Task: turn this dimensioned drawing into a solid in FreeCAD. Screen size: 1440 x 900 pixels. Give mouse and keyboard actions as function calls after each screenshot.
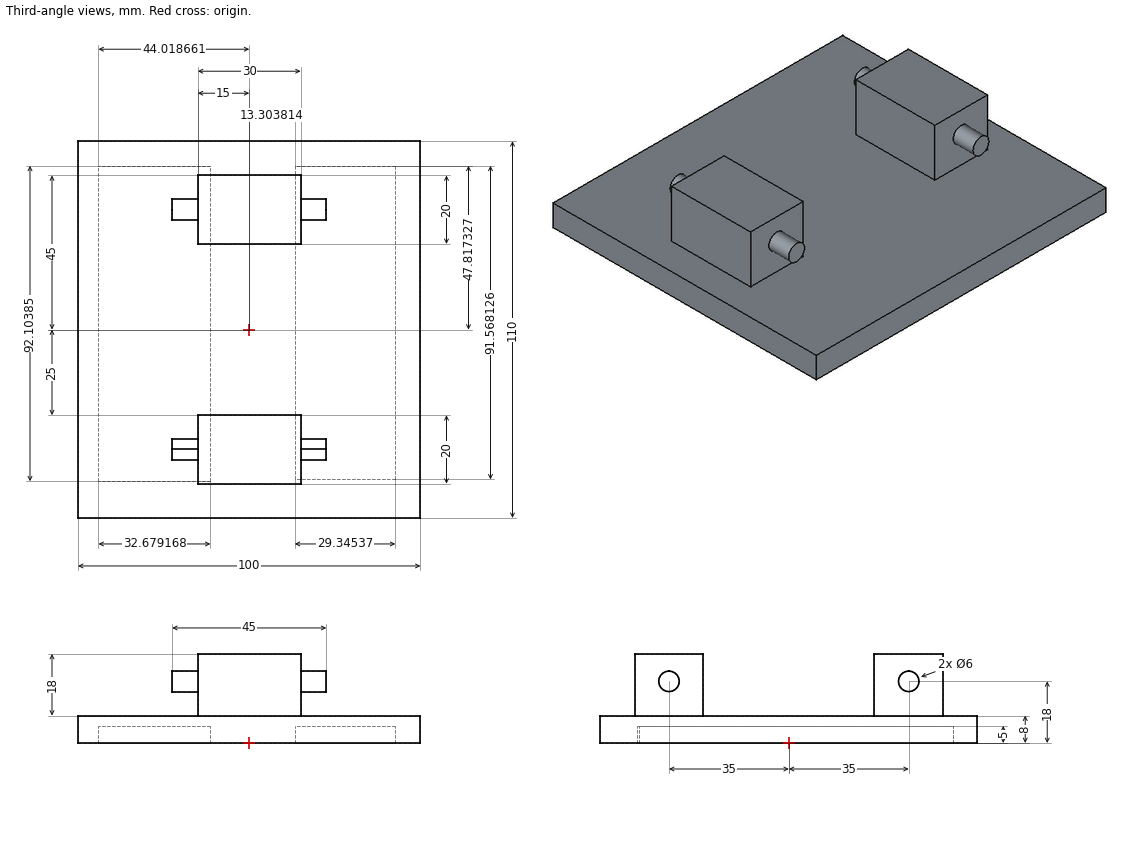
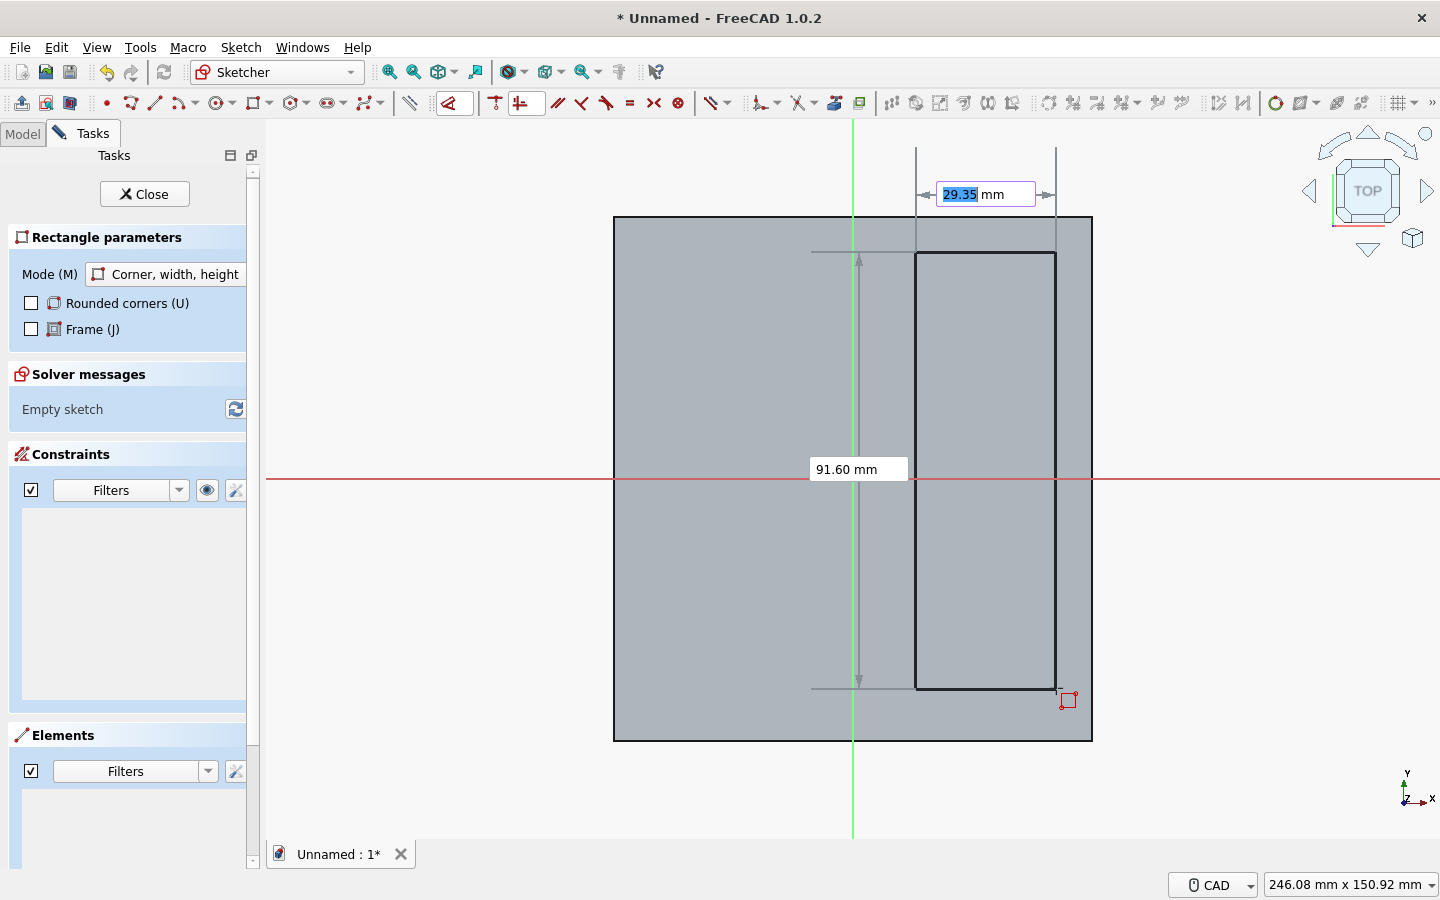
text(29.34537)
key(Tab)
text(91.568126)
key(Return)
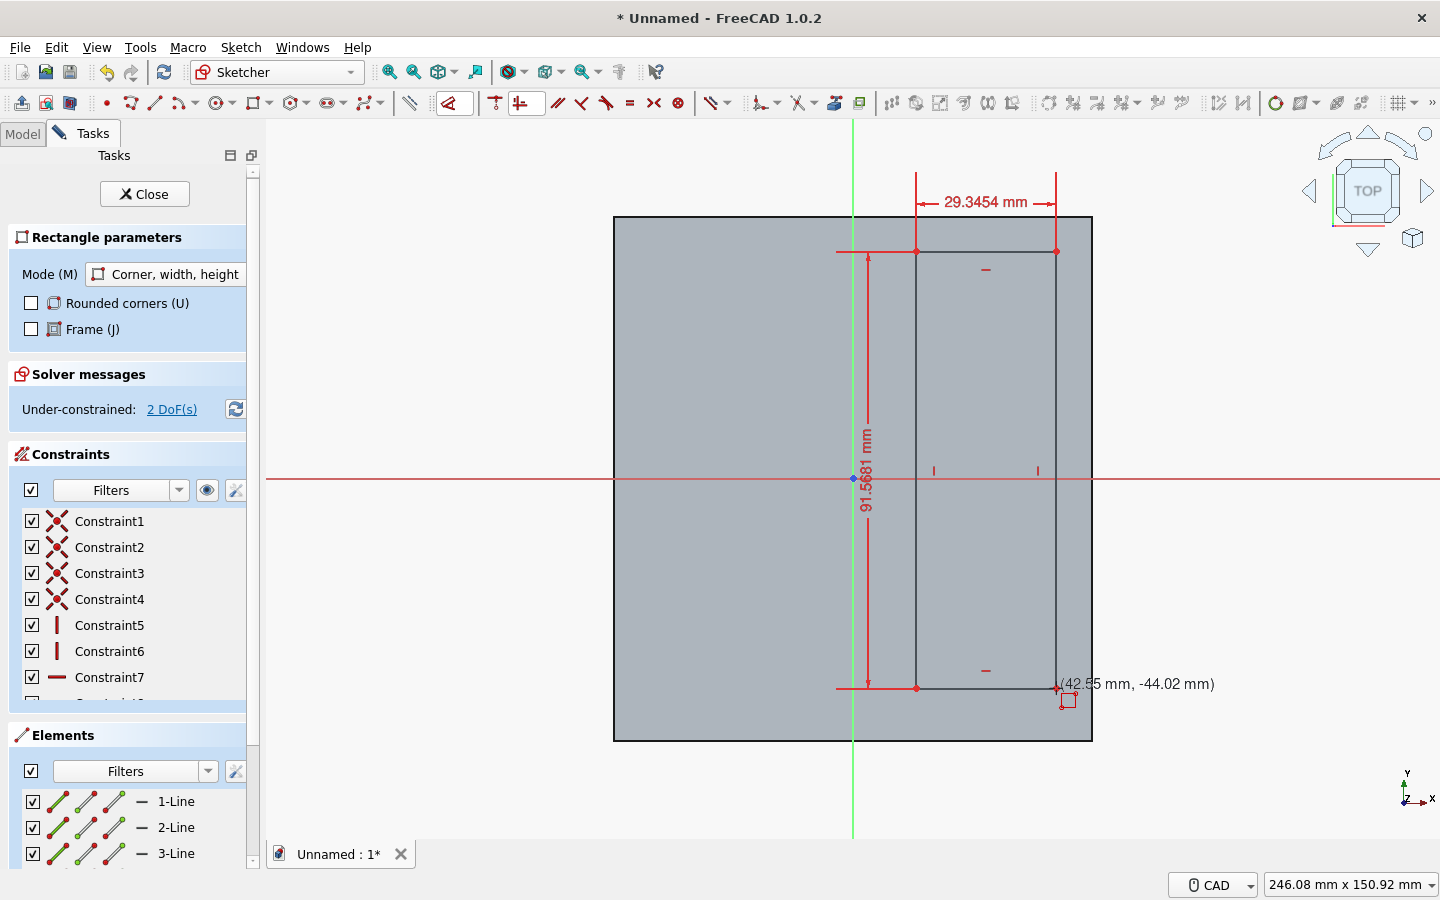
click(643, 251)
move(799, 690)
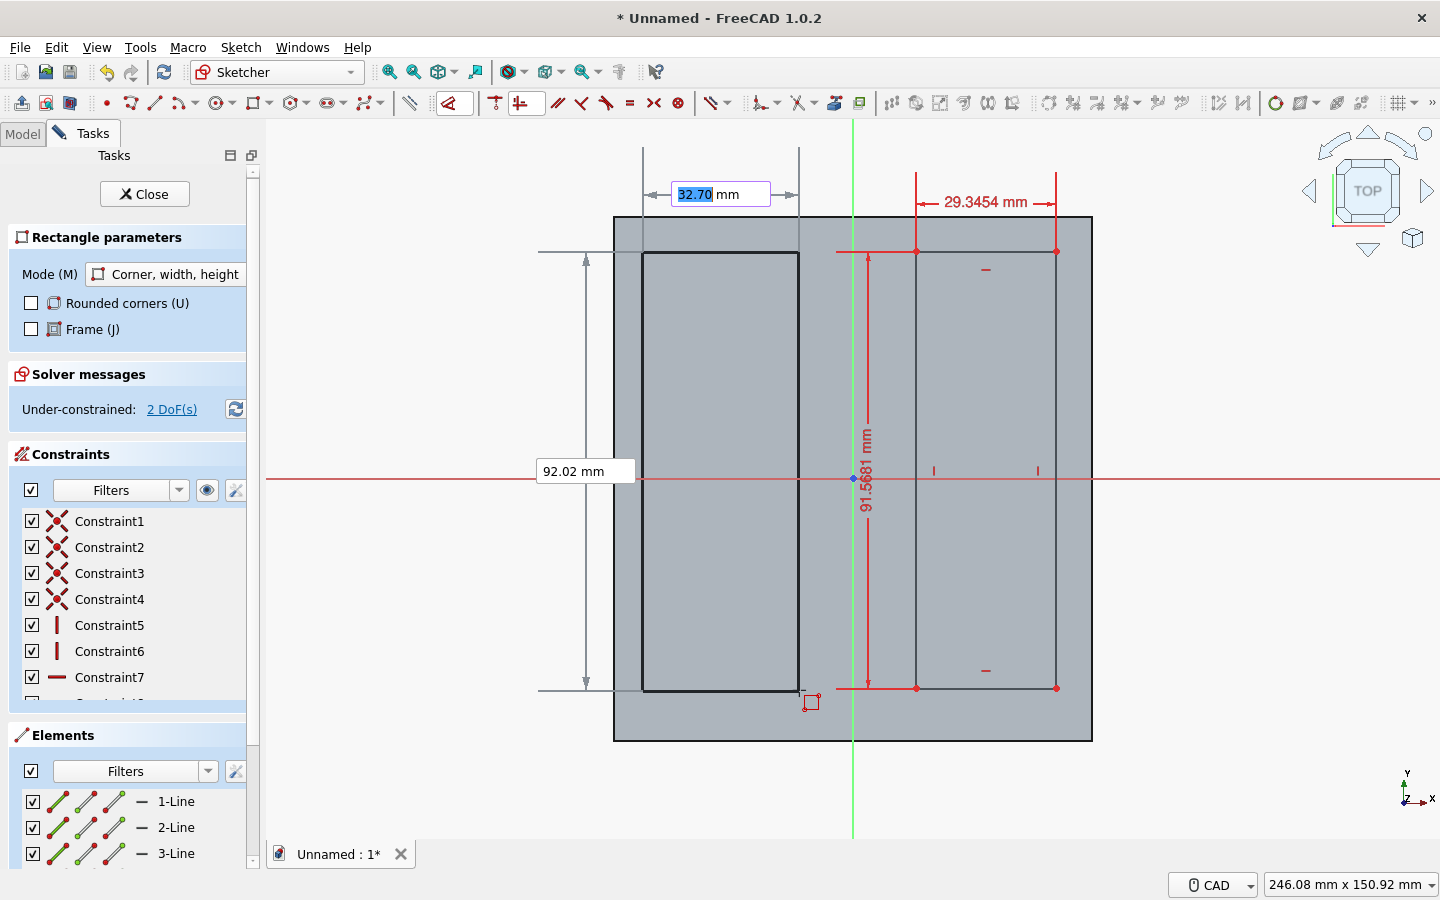
text(32.679168)
key(Tab)
text(92.10385)
key(Return)
key(Escape)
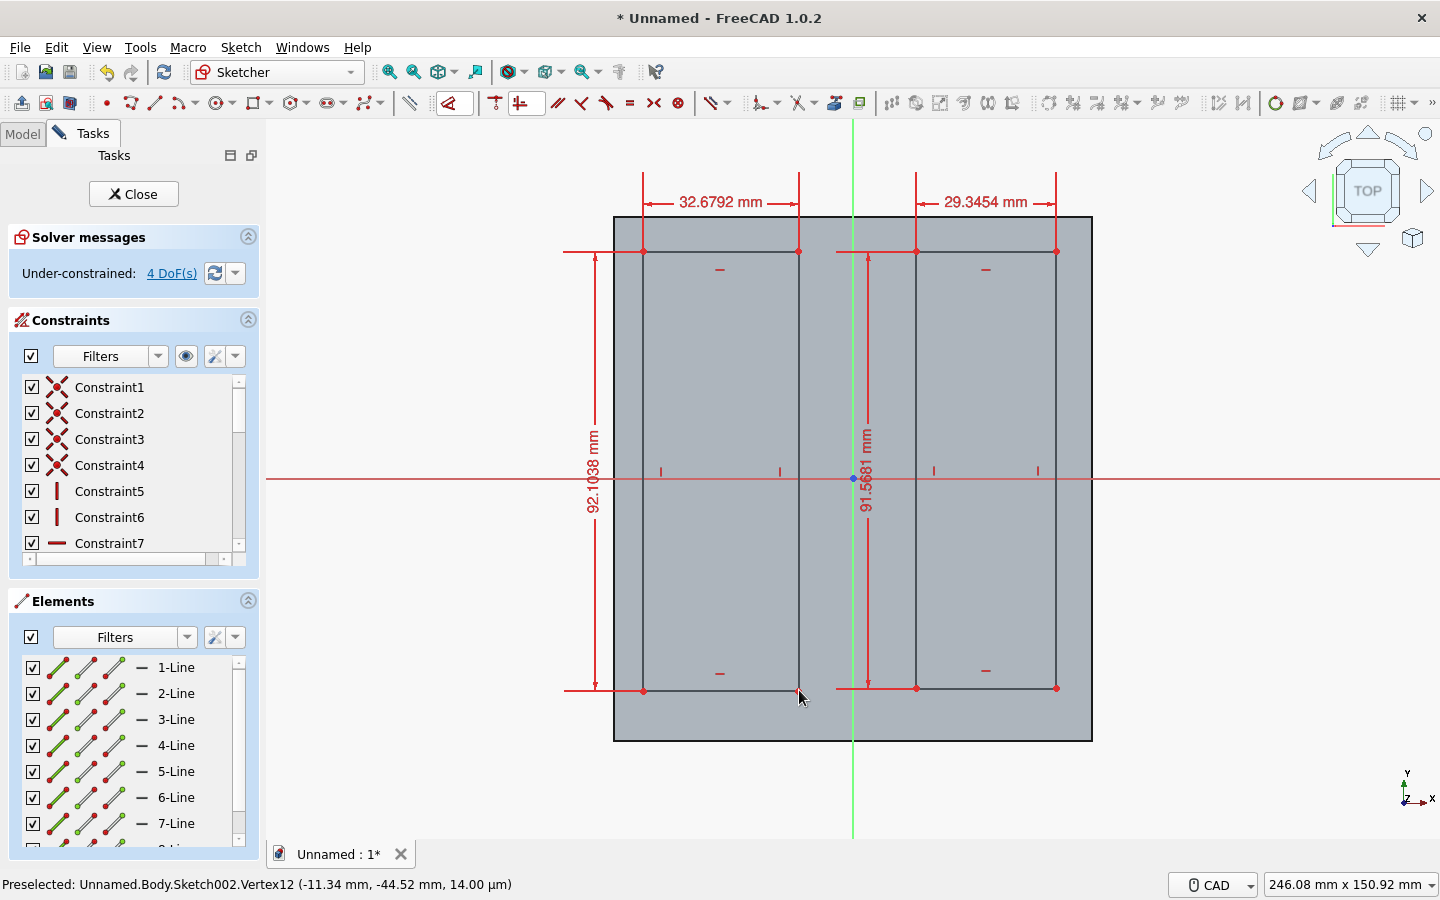
key(d)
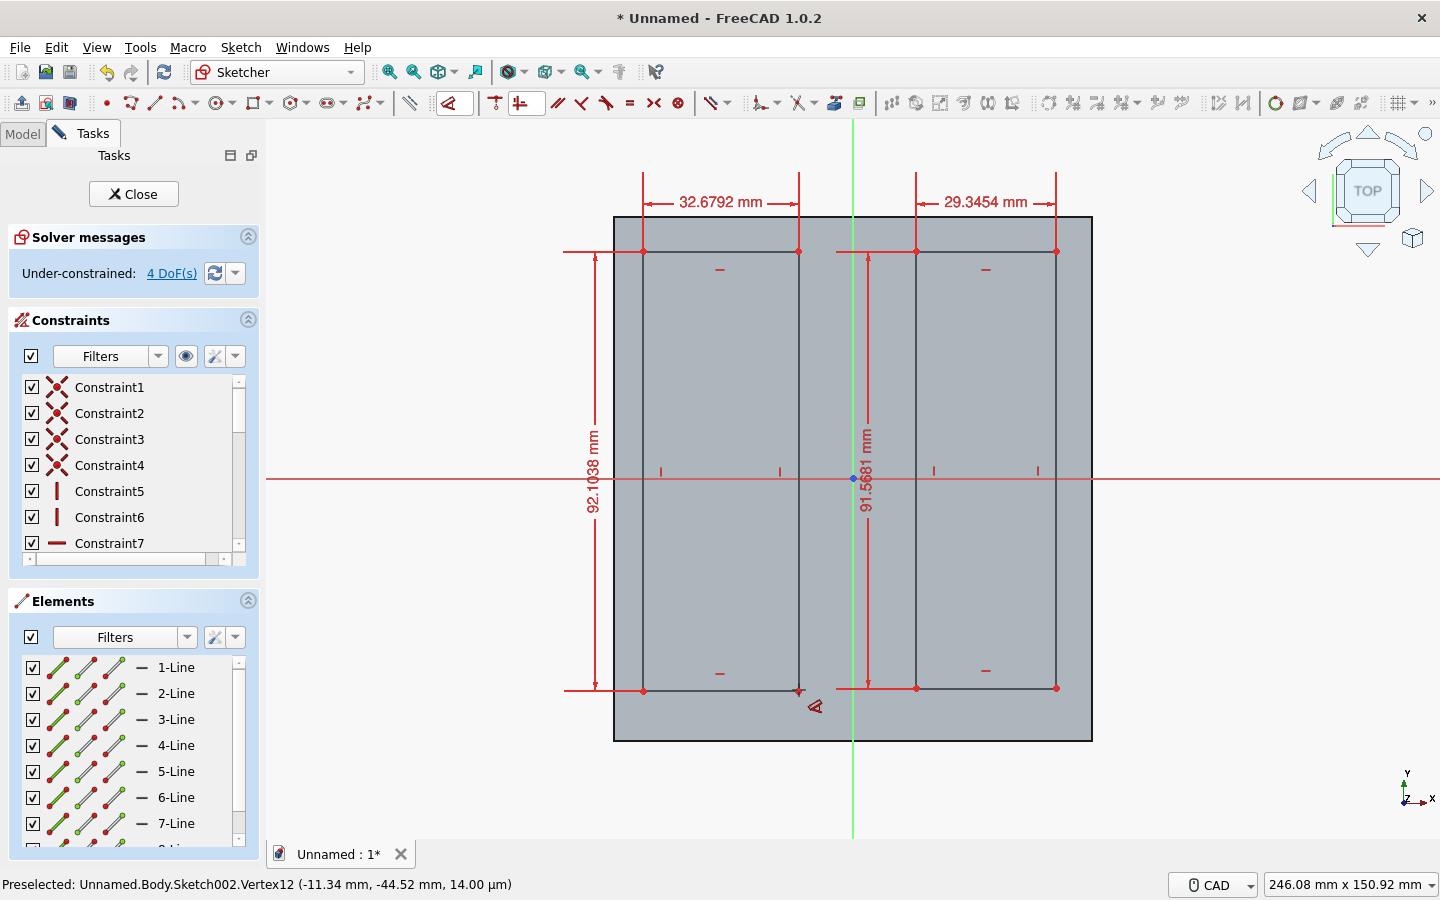
click(916, 252)
click(885, 218)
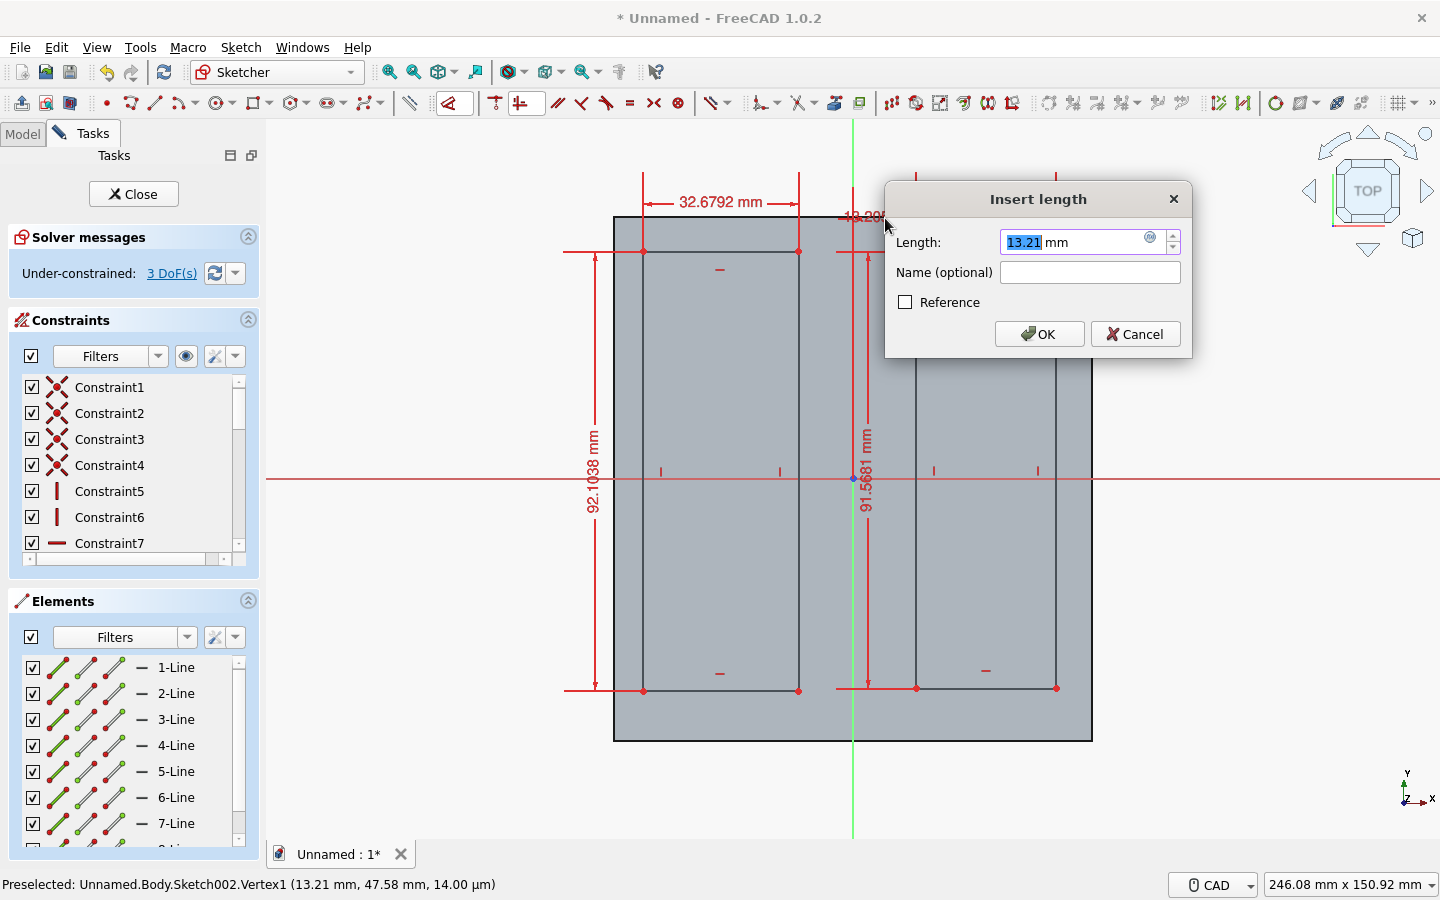
text(13.303814)
key(Return)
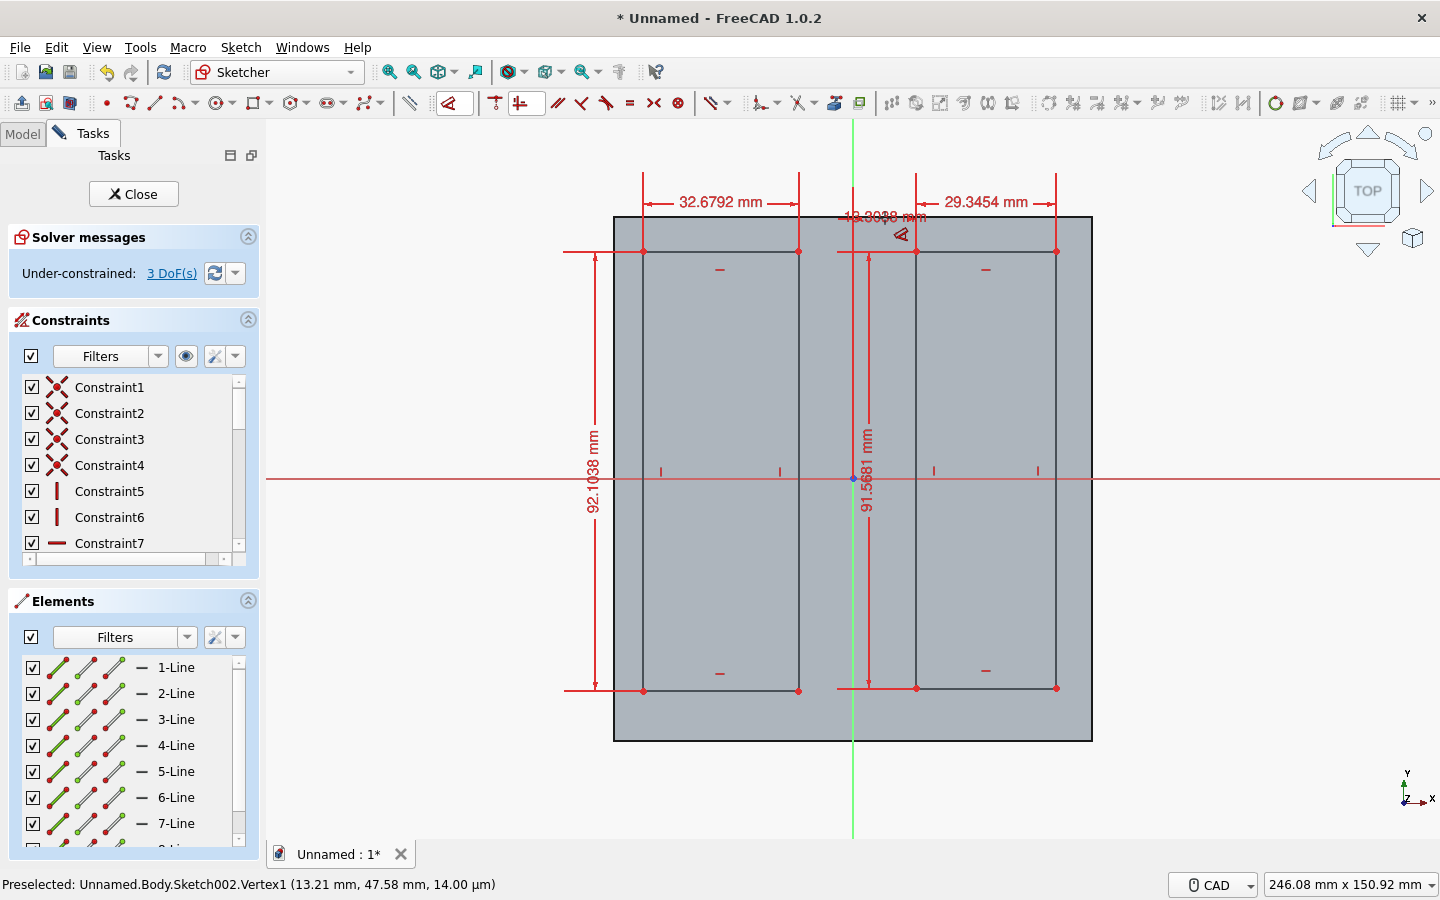
click(916, 252)
click(950, 366)